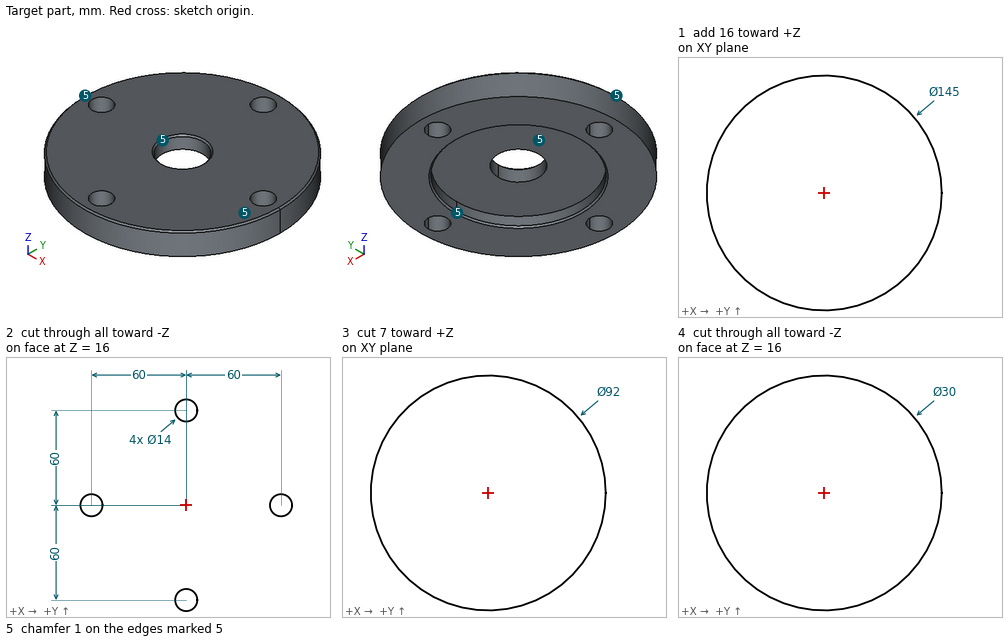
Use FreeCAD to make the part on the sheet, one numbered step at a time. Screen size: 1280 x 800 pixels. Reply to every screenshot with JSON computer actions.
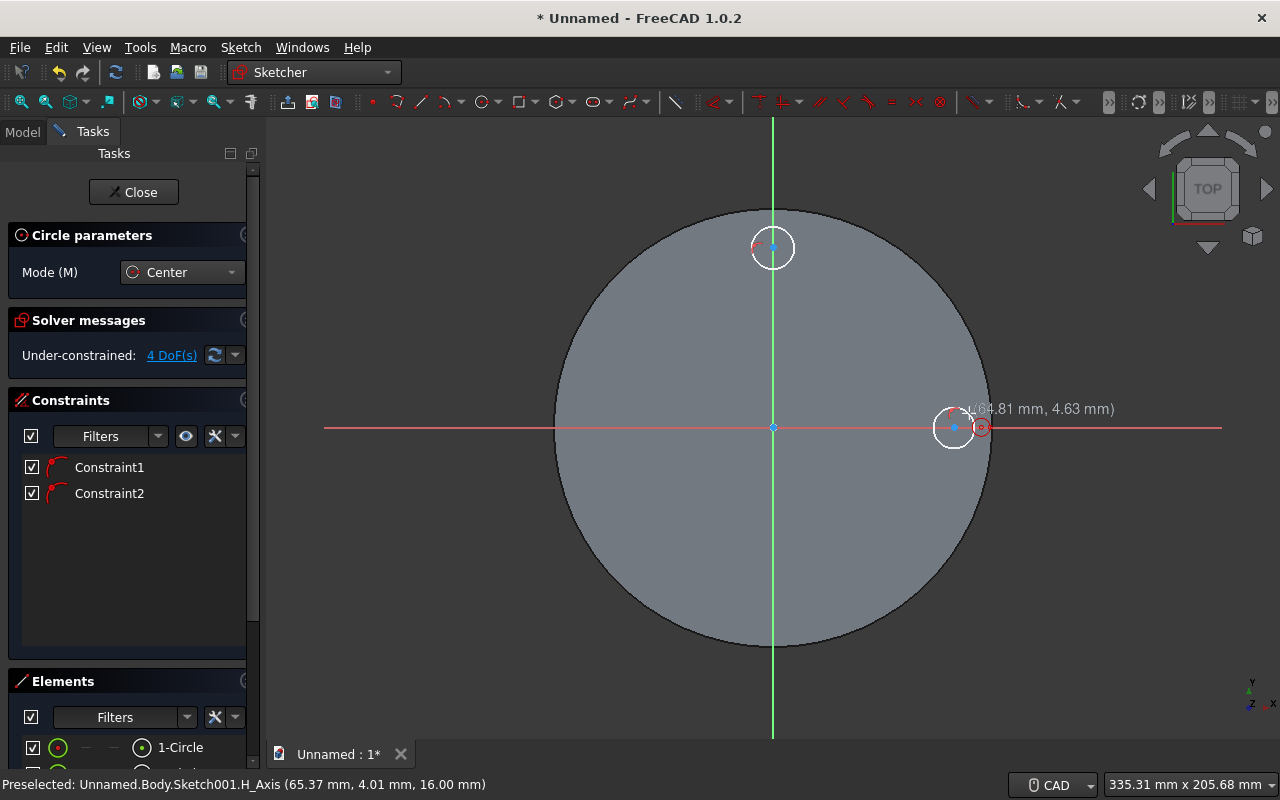
{"action": "left_click", "coordinate": [773, 609]}
{"action": "left_click", "coordinate": [788, 594]}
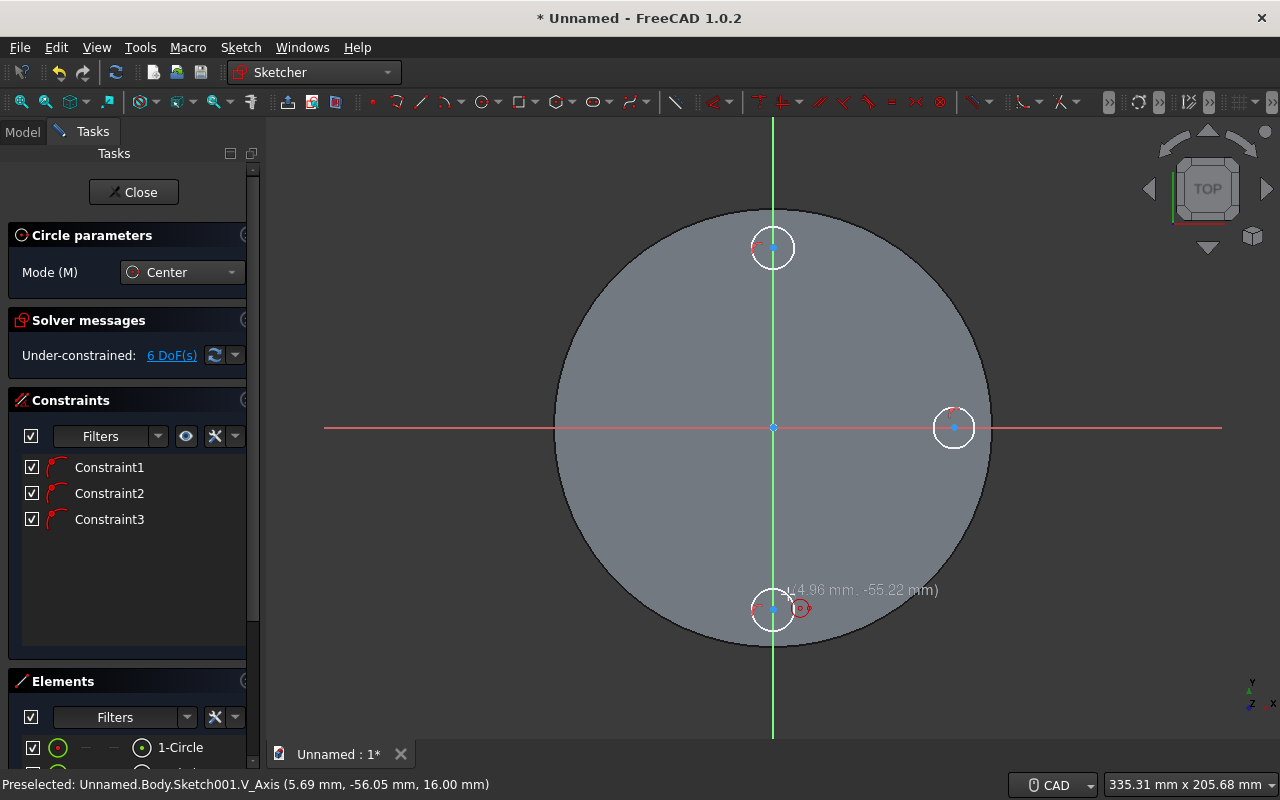
{"action": "left_click", "coordinate": [592, 428]}
{"action": "left_click", "coordinate": [607, 413]}
{"action": "key", "text": "Escape"}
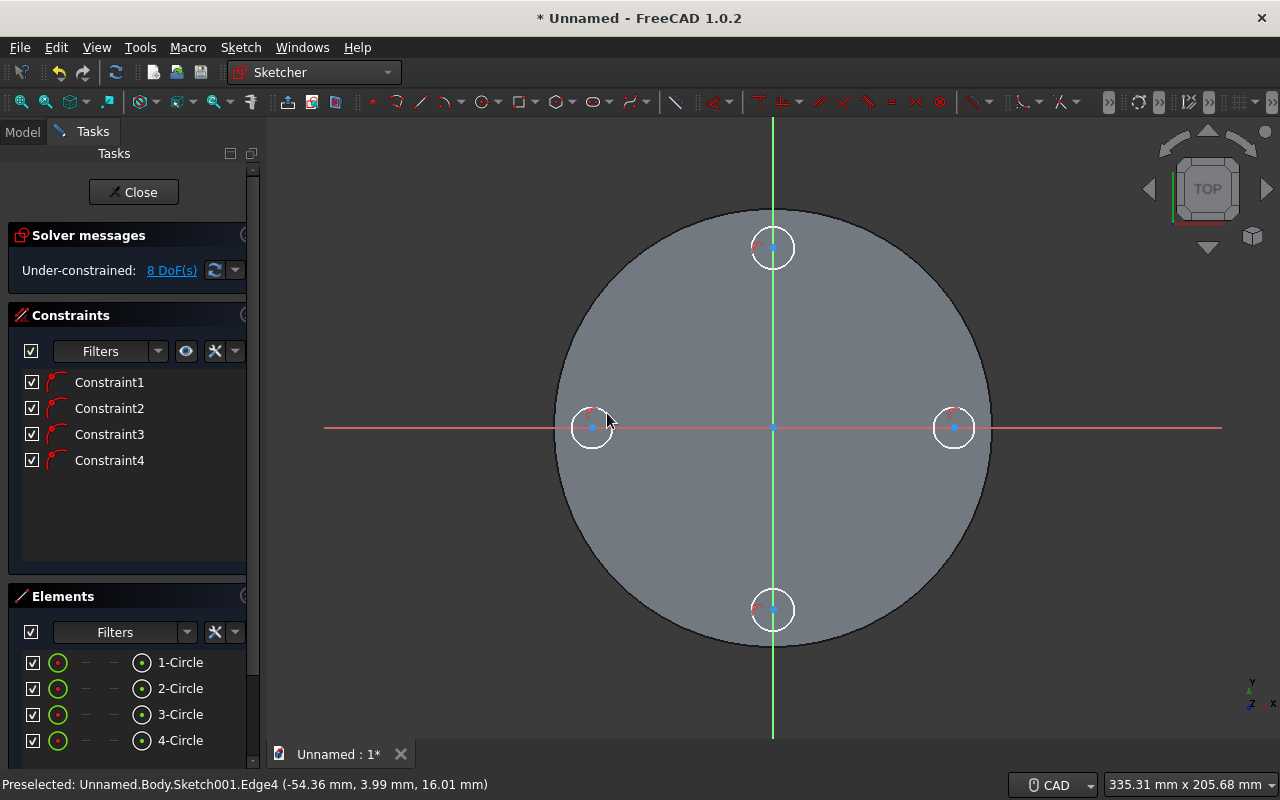
{"action": "left_click", "coordinate": [788, 233]}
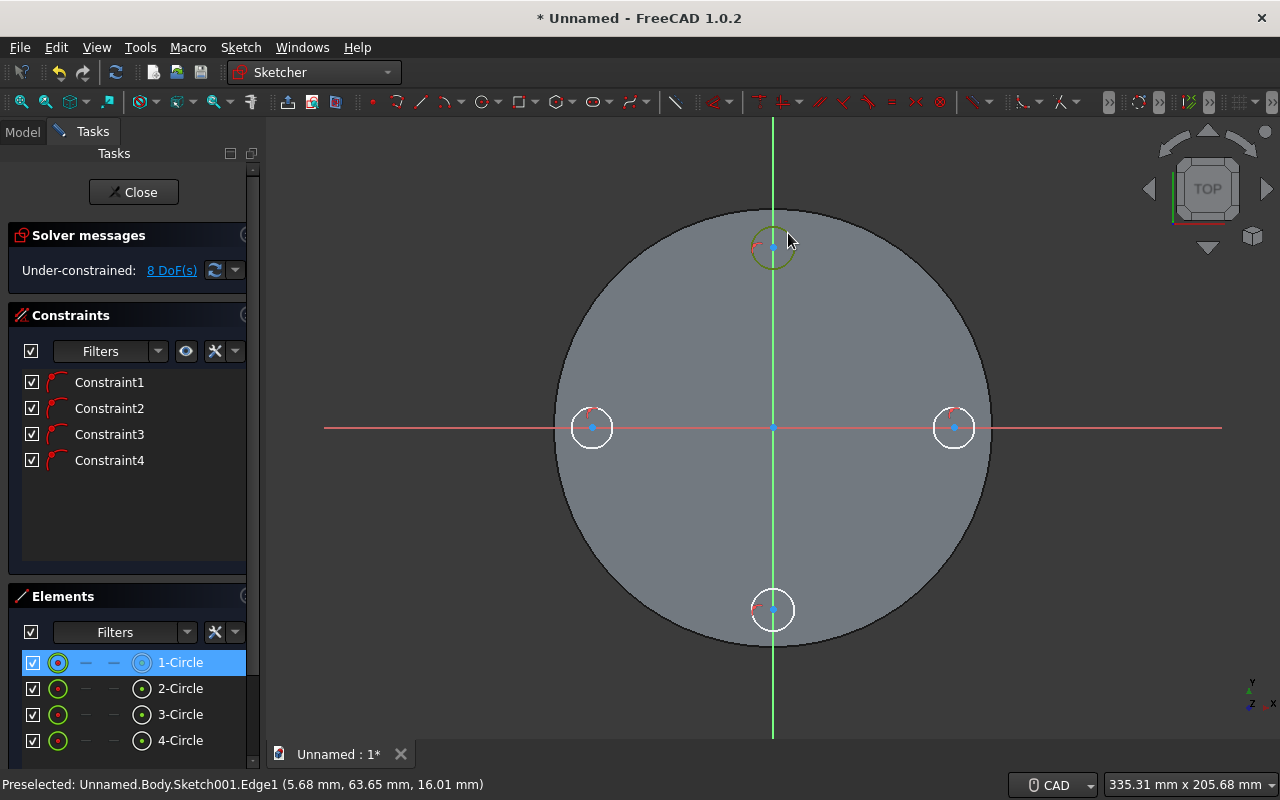
{"action": "left_click", "coordinate": [968, 413]}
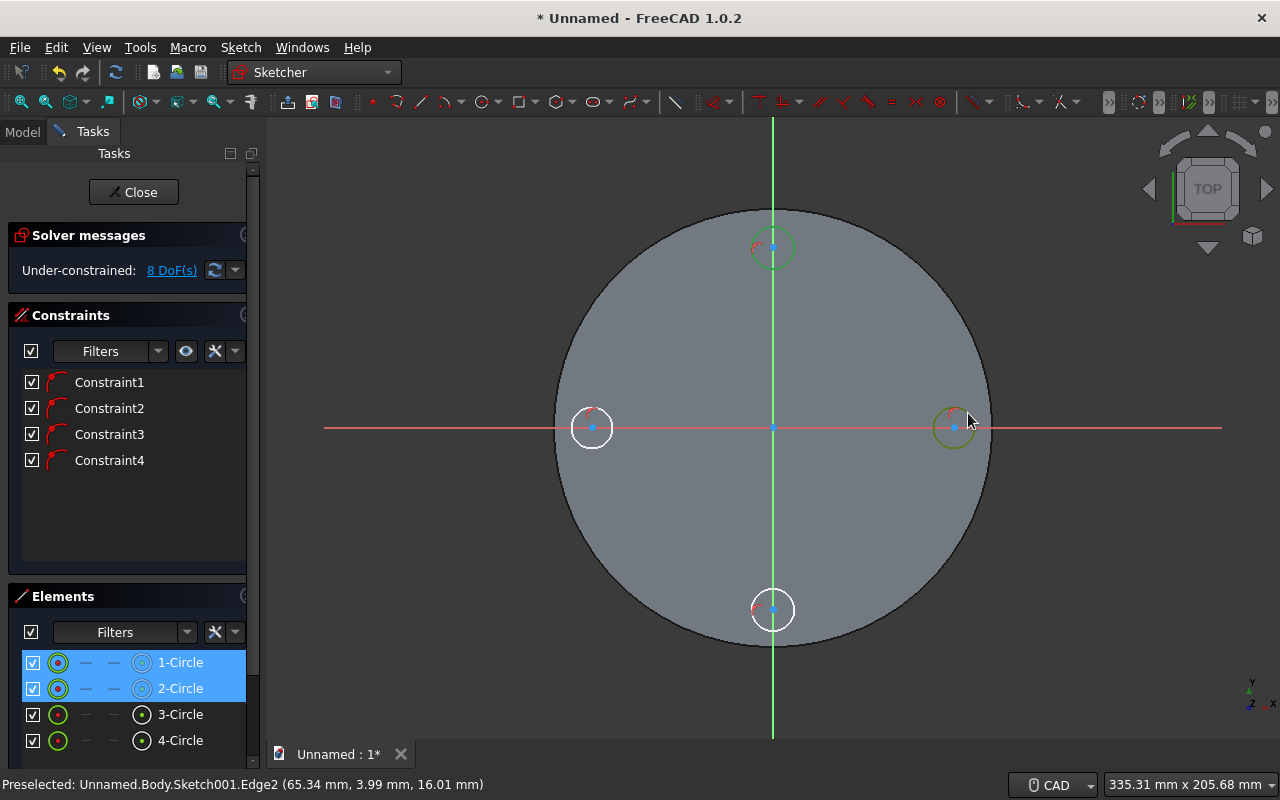
{"action": "left_click", "coordinate": [788, 595]}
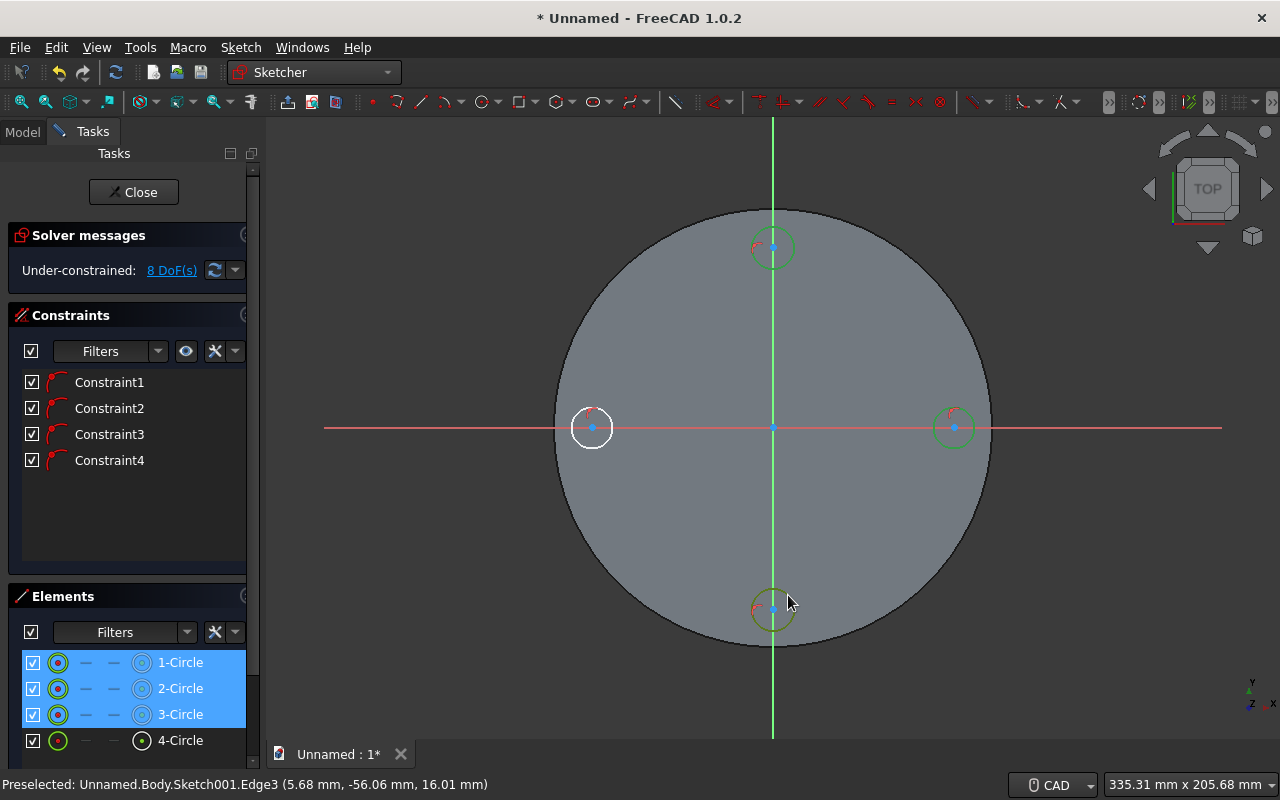
{"action": "left_click", "coordinate": [606, 413]}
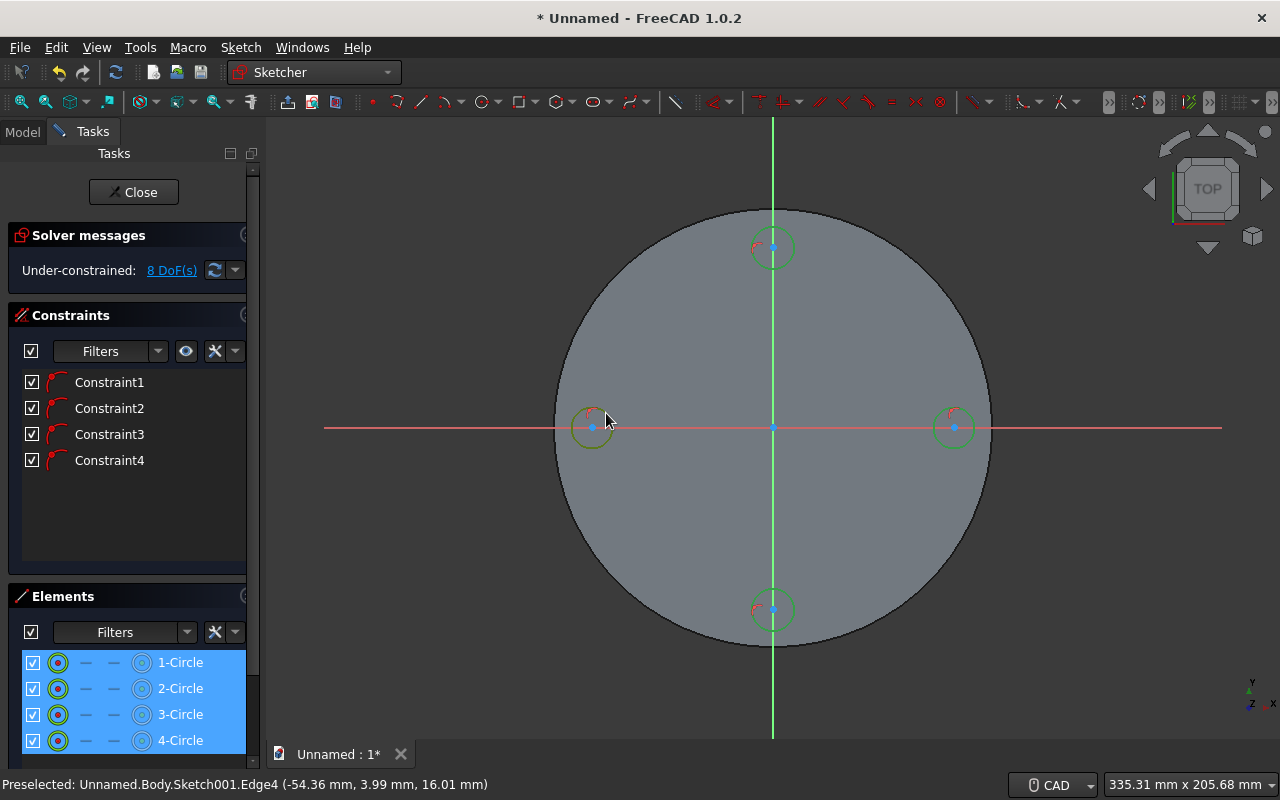
{"action": "left_click", "coordinate": [892, 102]}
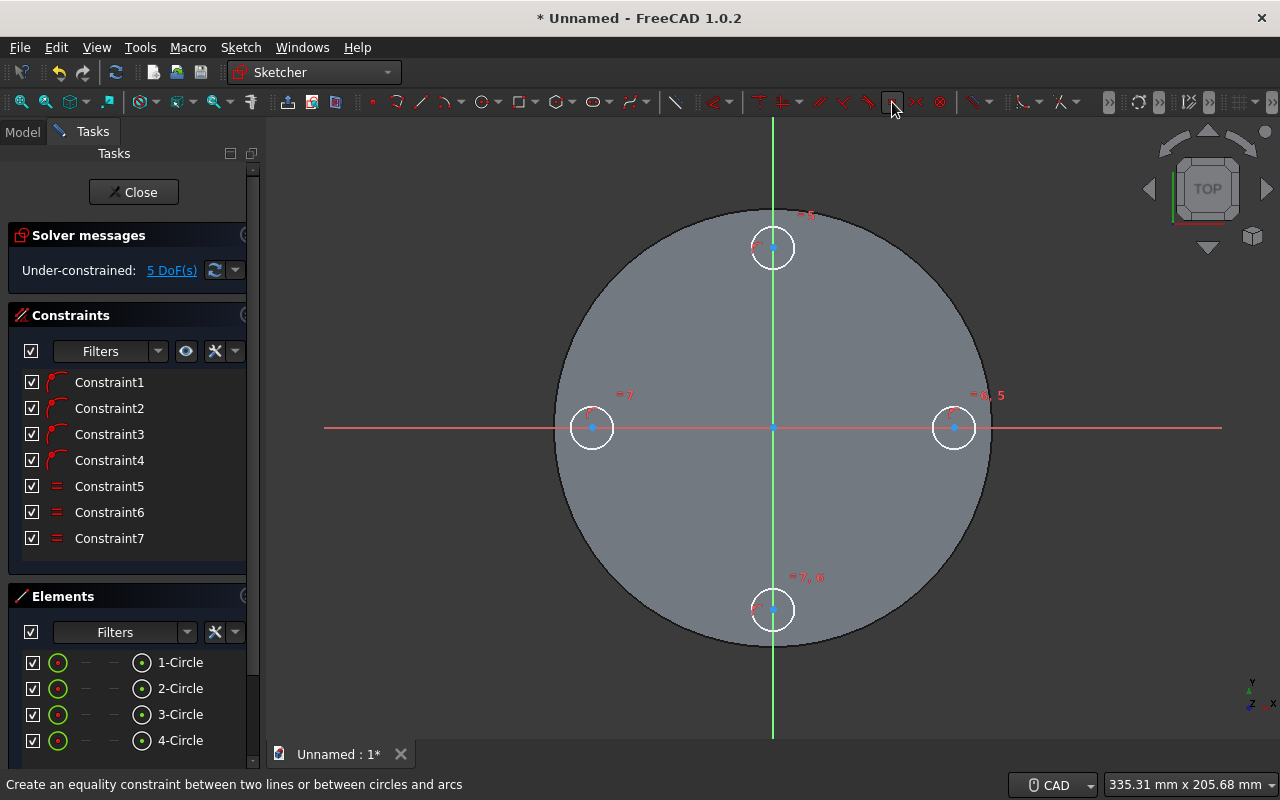
{"action": "key", "text": "d"}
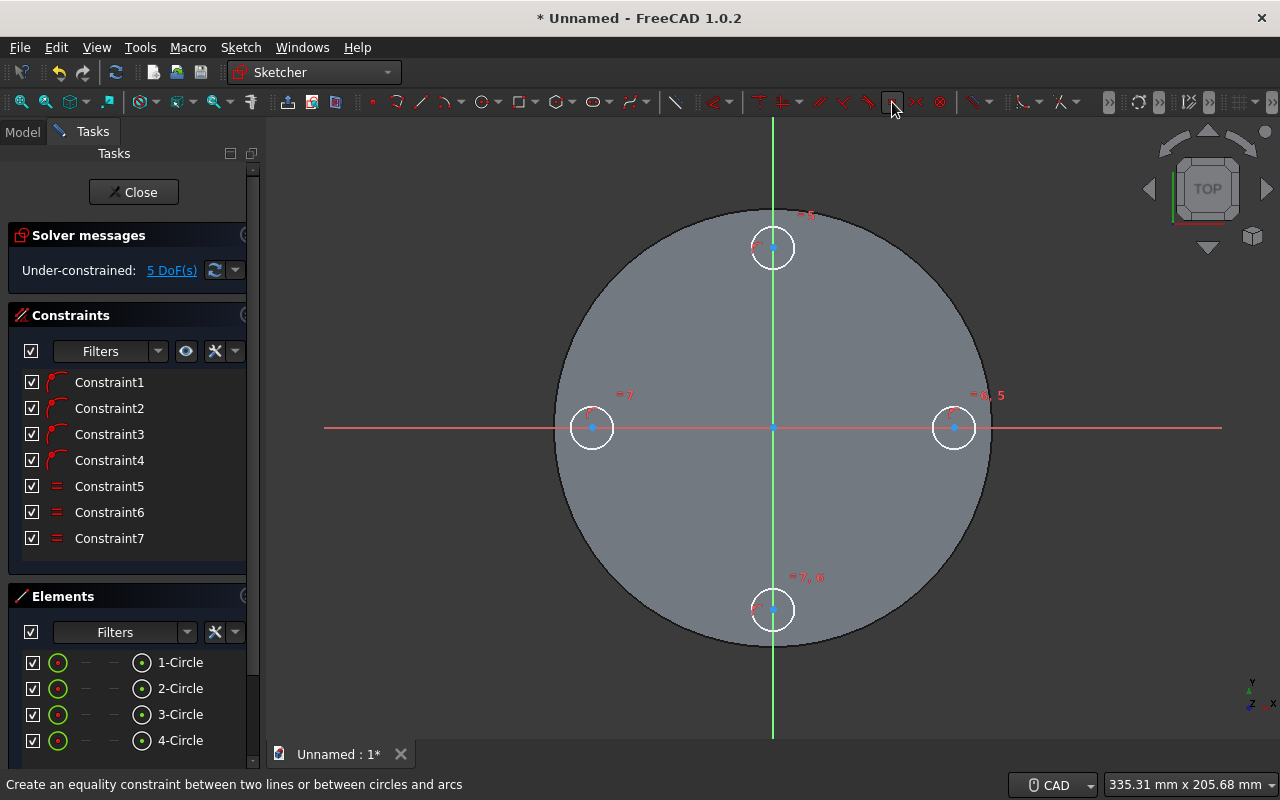
{"action": "left_click", "coordinate": [788, 233]}
{"action": "left_click", "coordinate": [811, 210]}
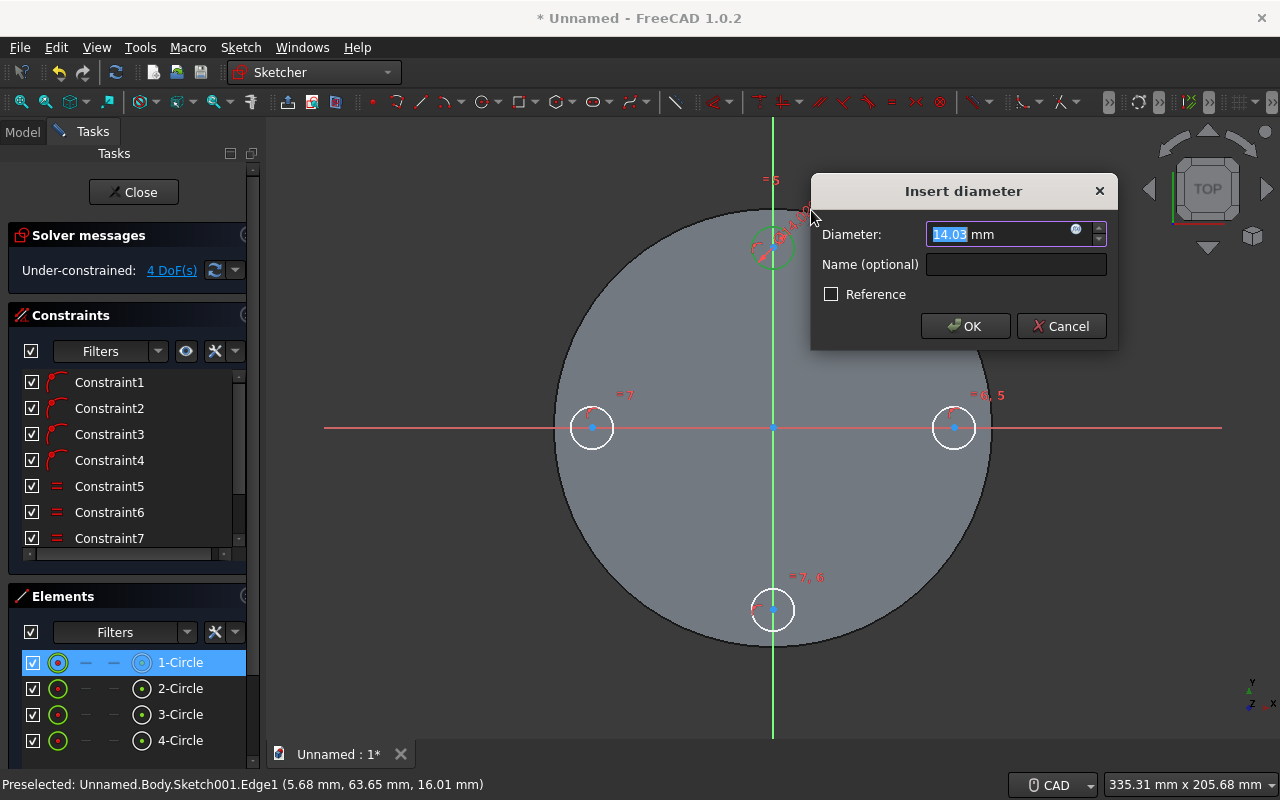
{"action": "type", "text": "14"}
{"action": "key", "text": "Return"}